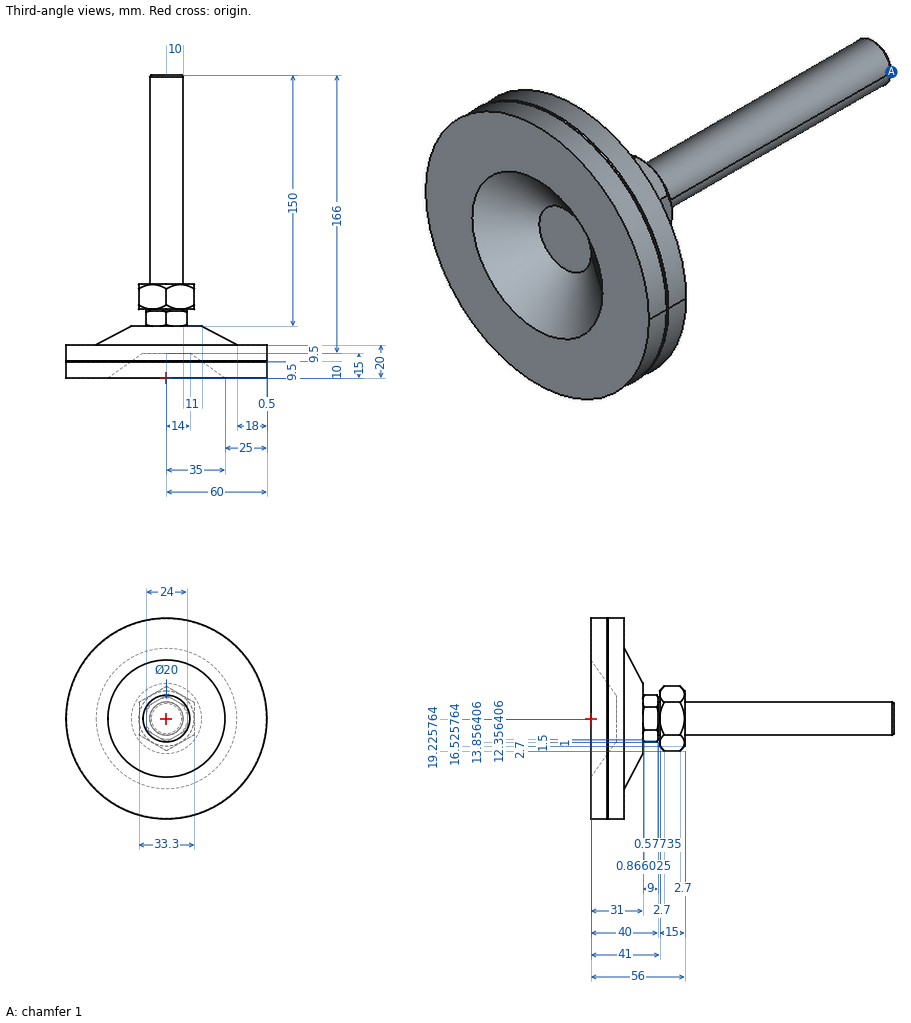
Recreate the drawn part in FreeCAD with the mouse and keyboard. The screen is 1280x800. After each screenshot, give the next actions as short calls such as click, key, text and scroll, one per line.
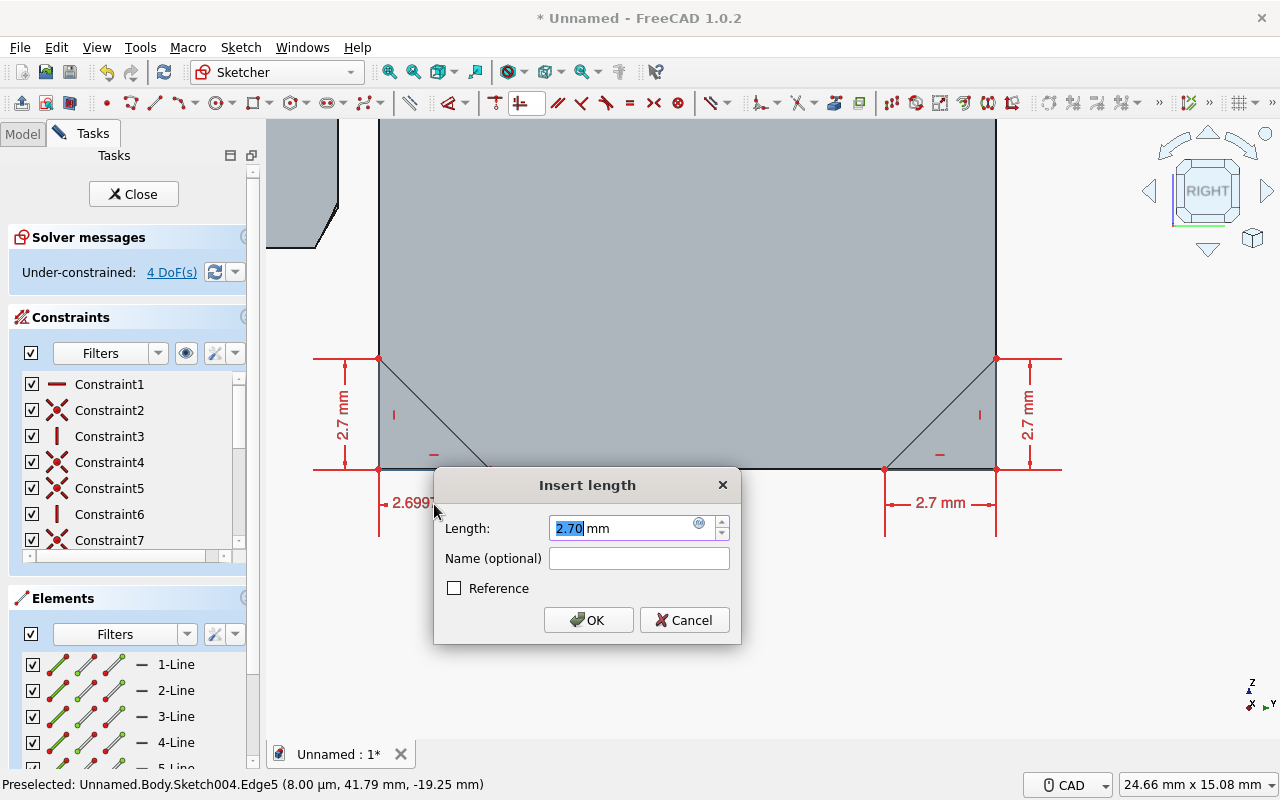
text(2.7)
key(Return)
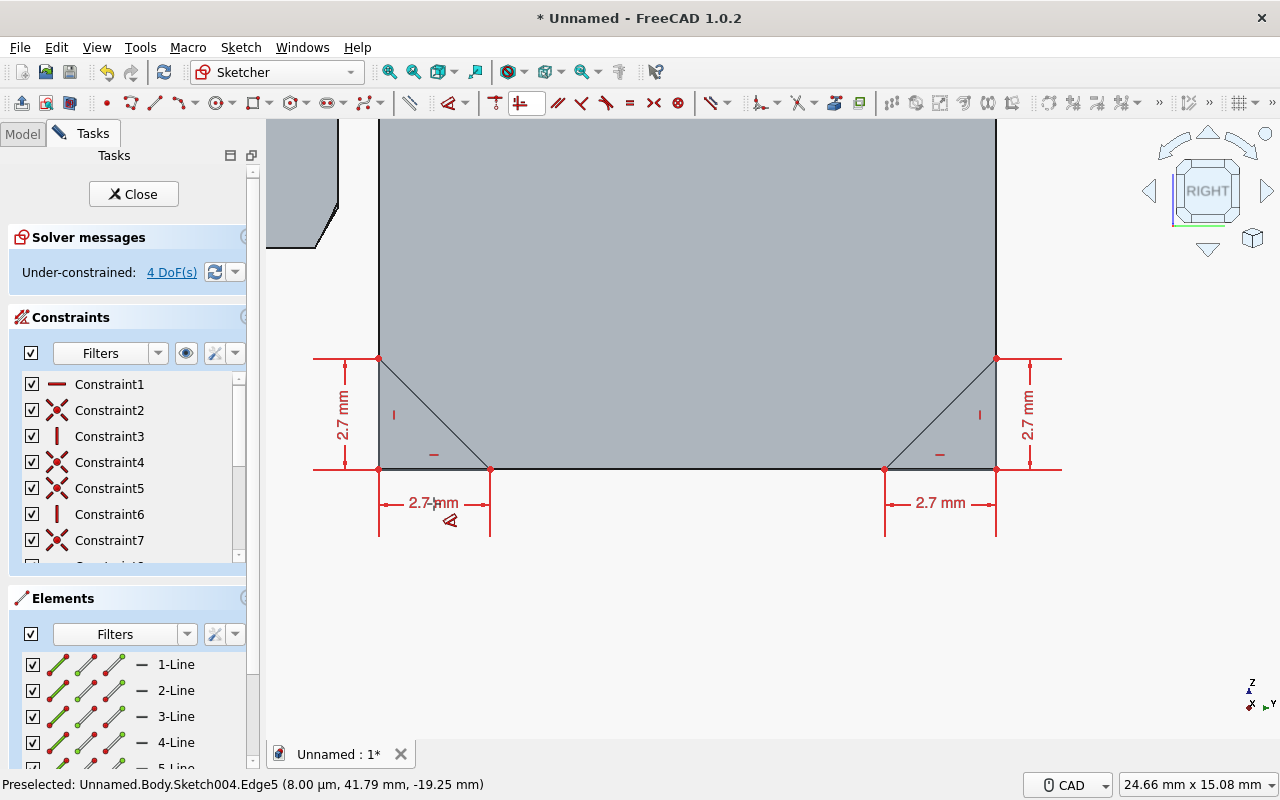
click(996, 470)
click(645, 504)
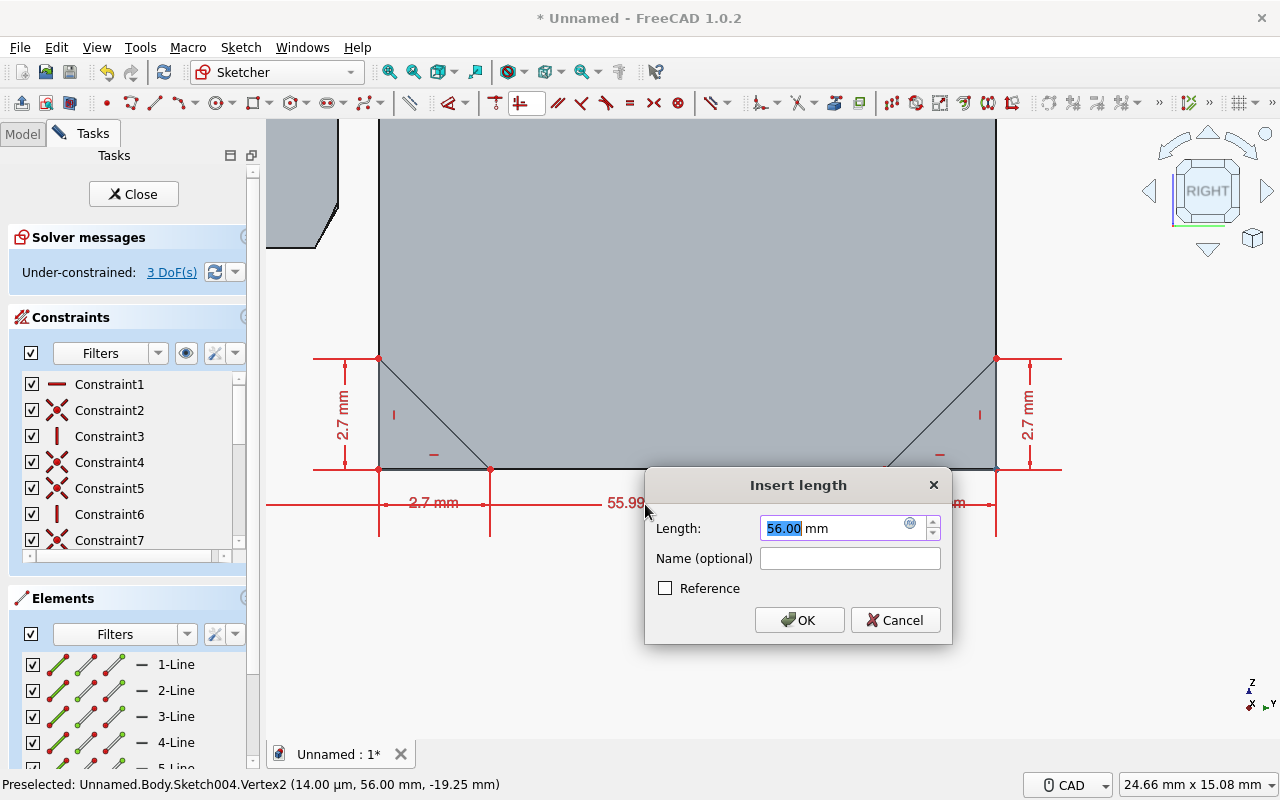
text(56)
key(Return)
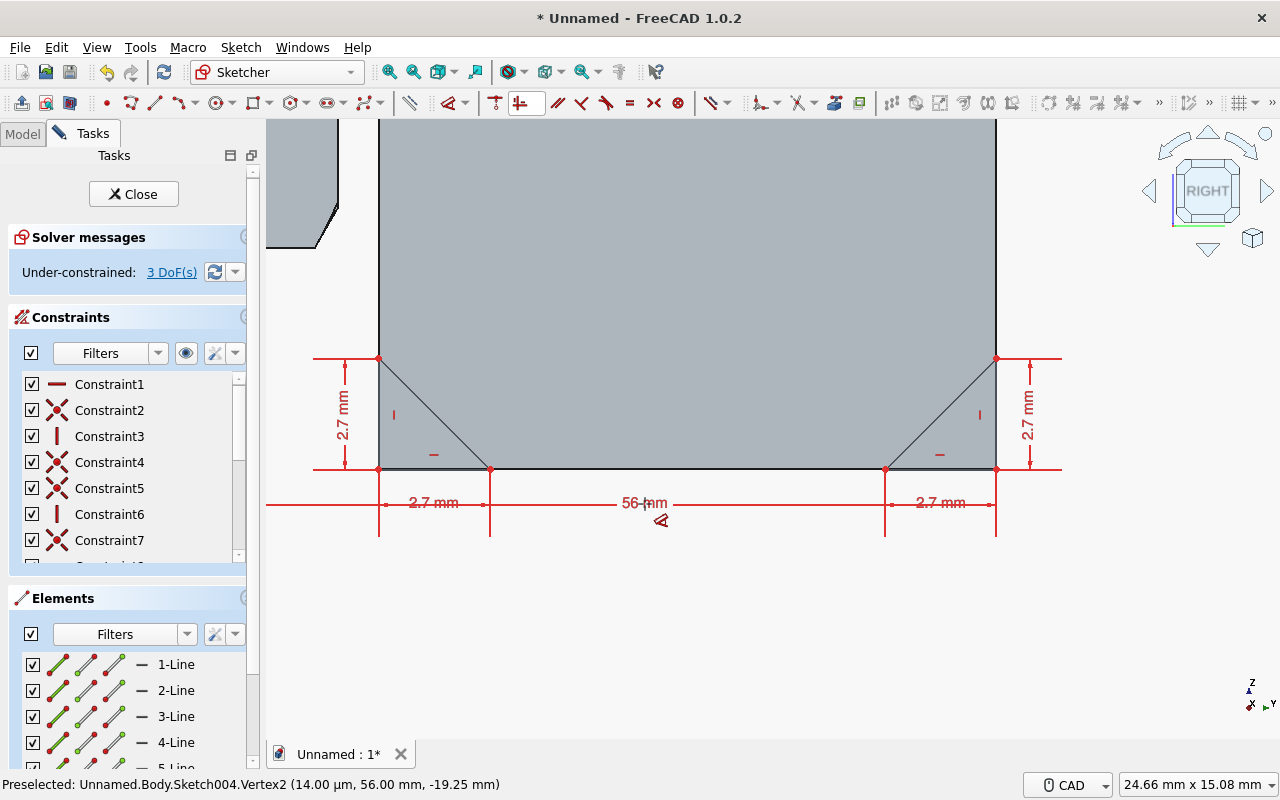
click(379, 359)
click(336, 393)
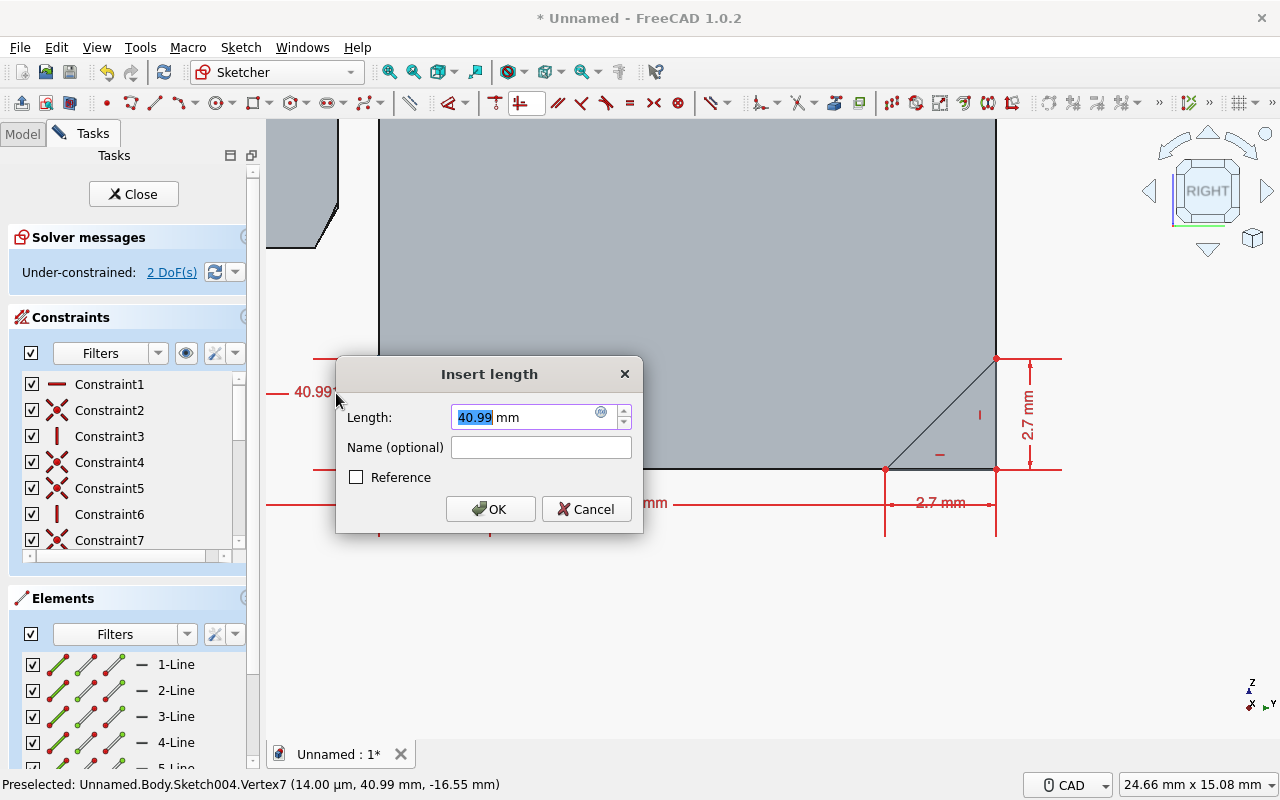
text(41)
key(Return)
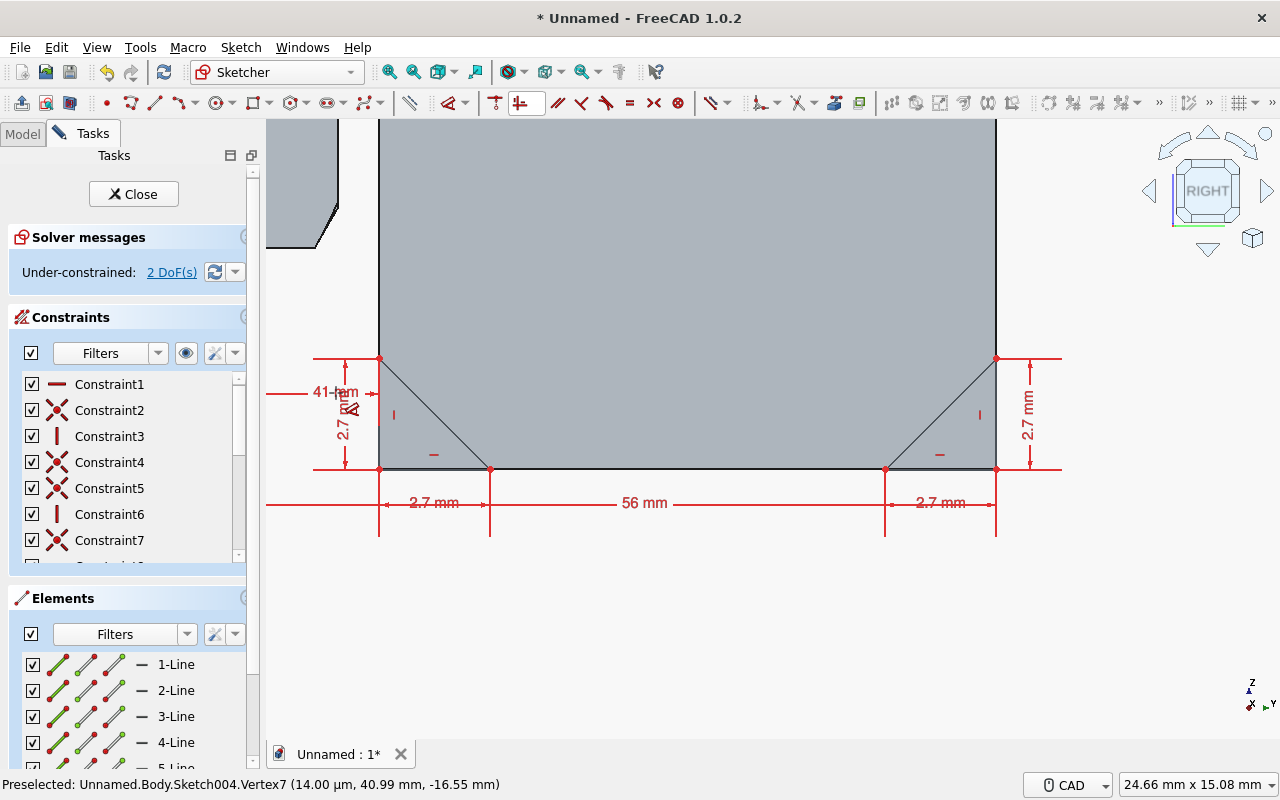
click(885, 470)
click(919, 309)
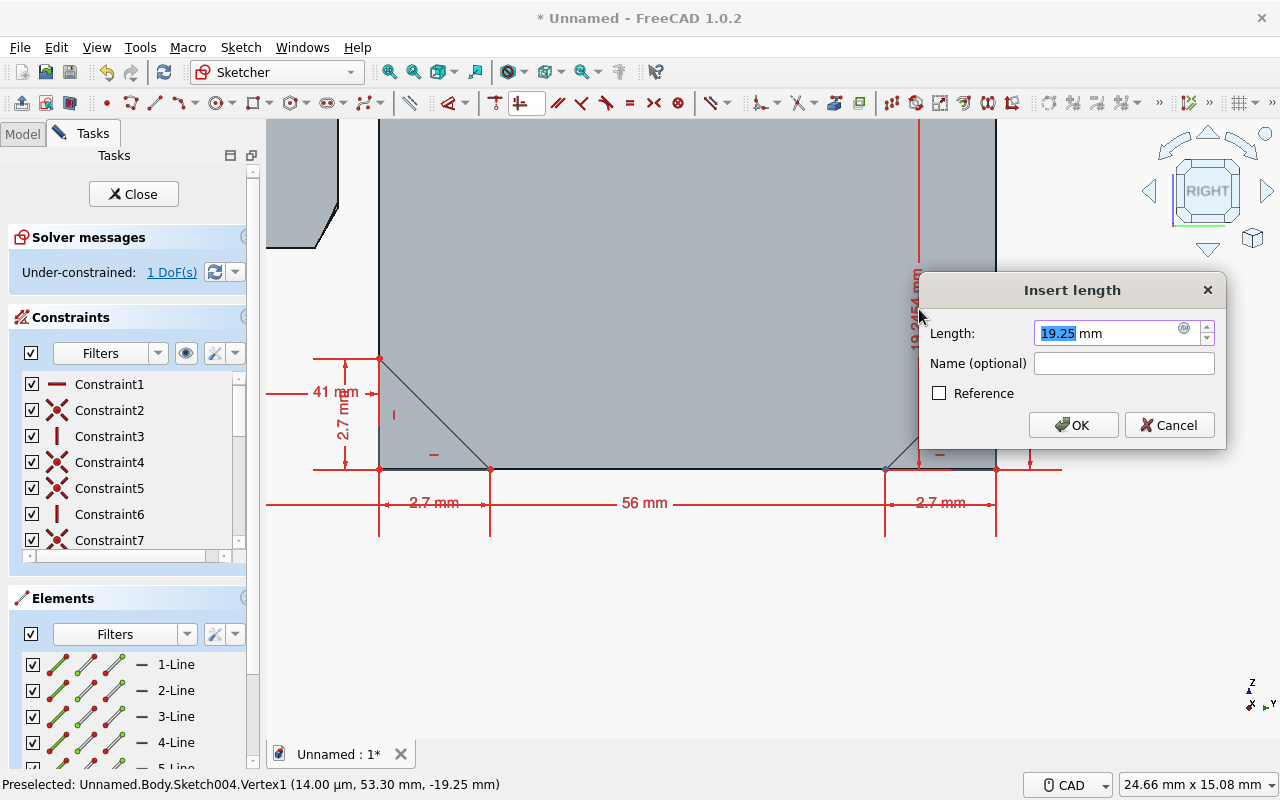
text(19.225764)
key(Return)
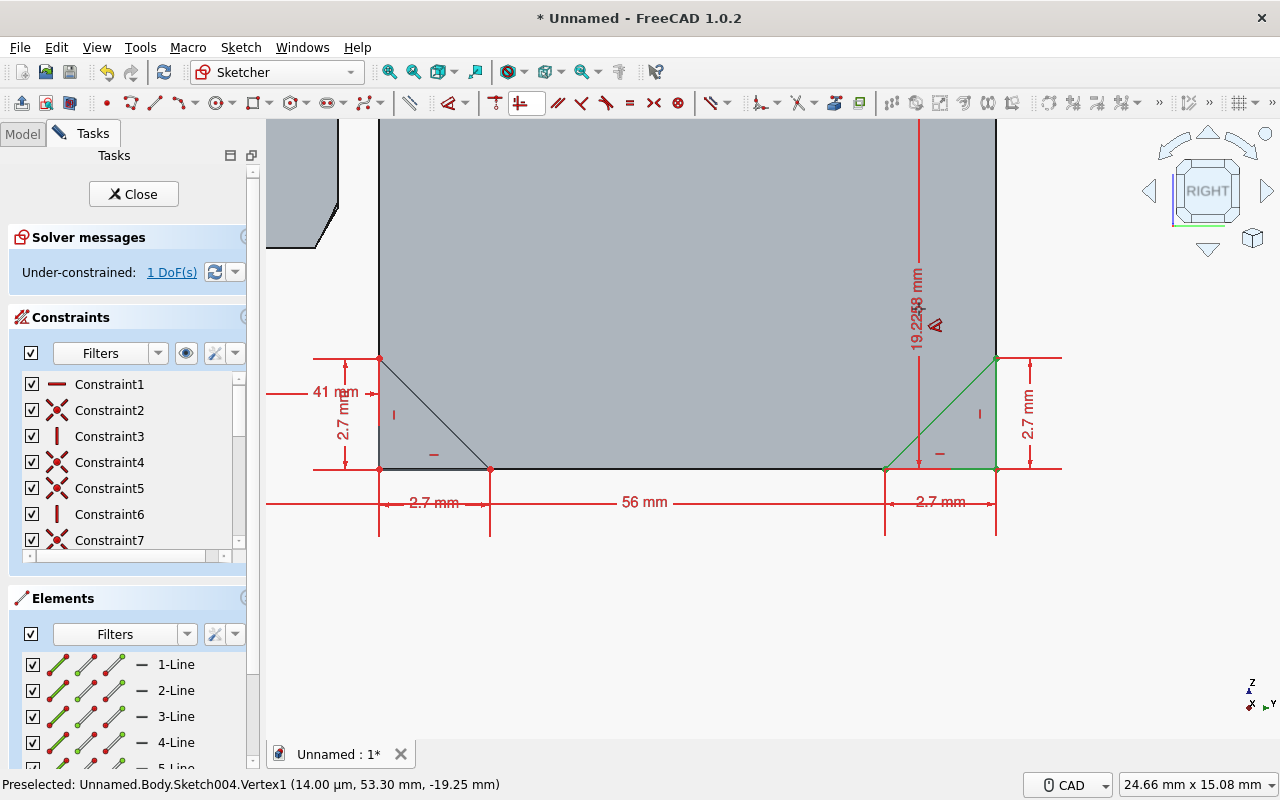
click(379, 359)
click(413, 253)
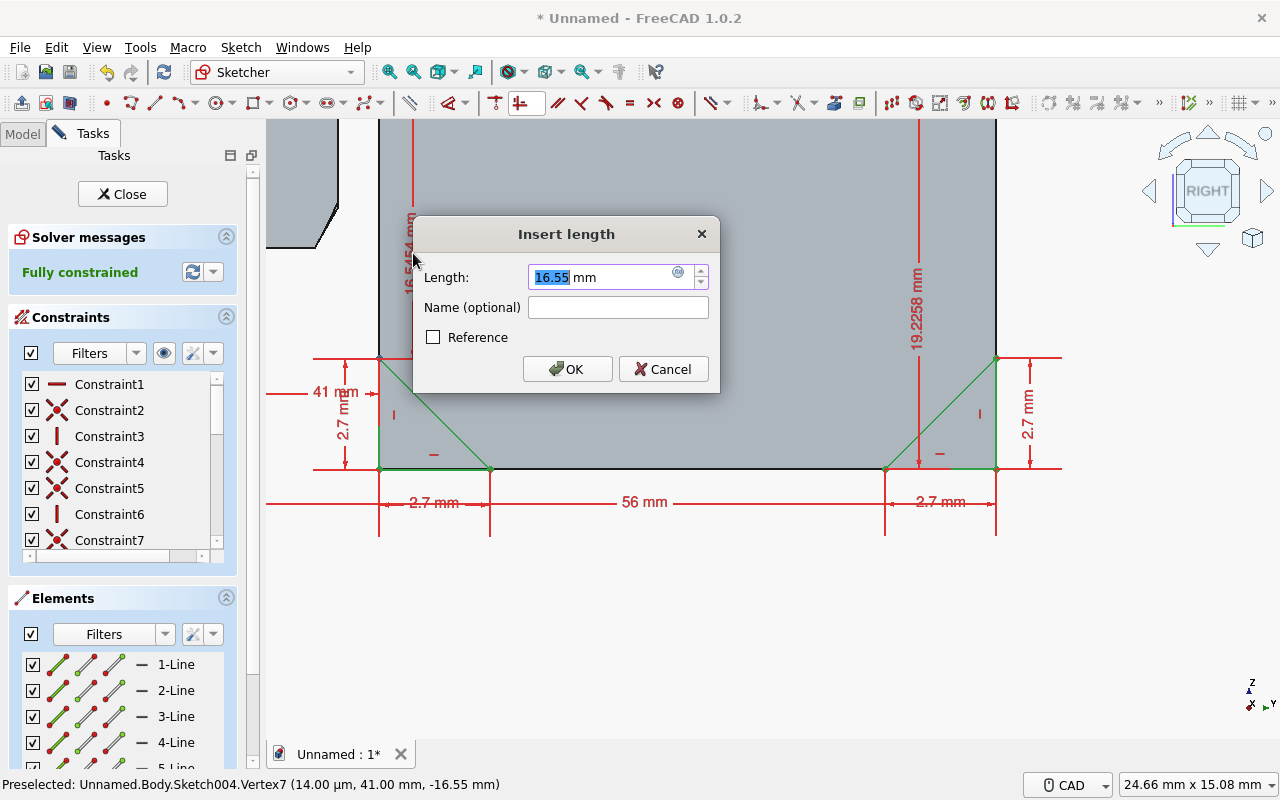
text(16.525764)
key(Return)
key(Escape)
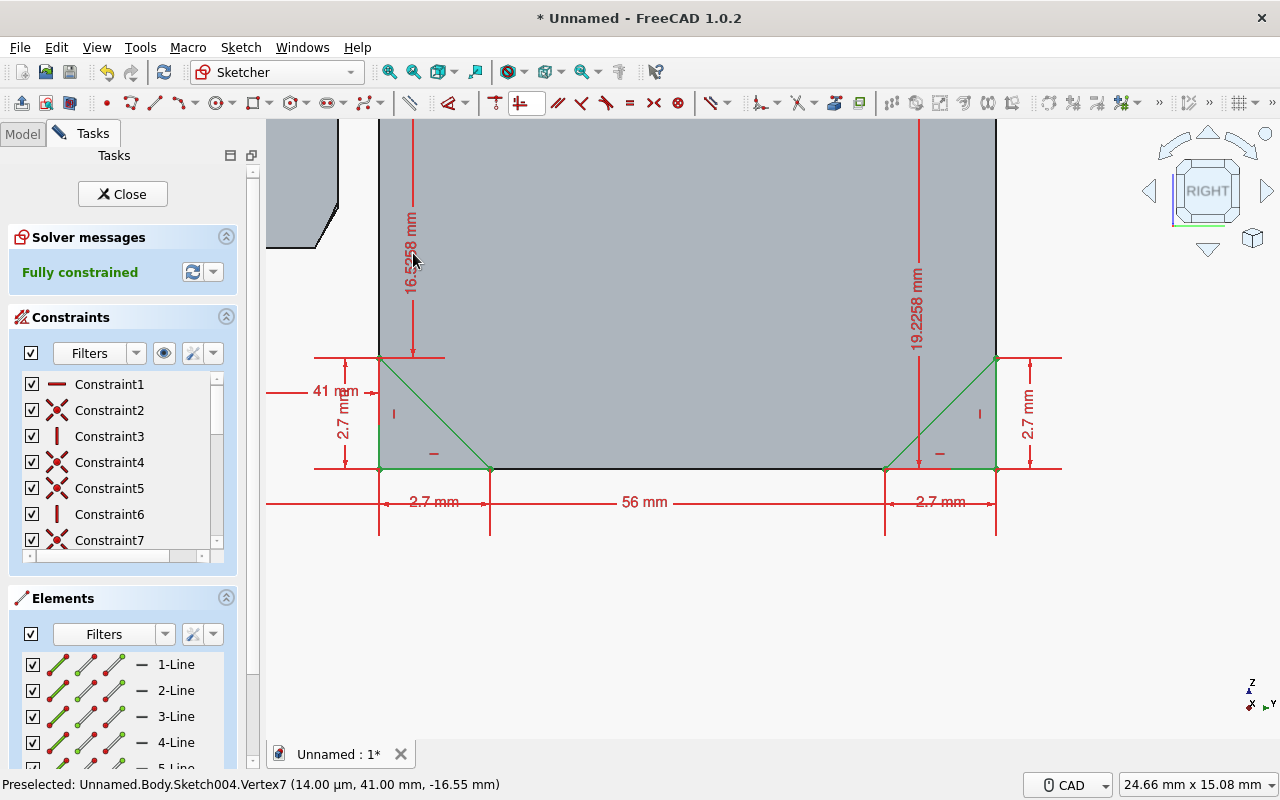
click(123, 194)